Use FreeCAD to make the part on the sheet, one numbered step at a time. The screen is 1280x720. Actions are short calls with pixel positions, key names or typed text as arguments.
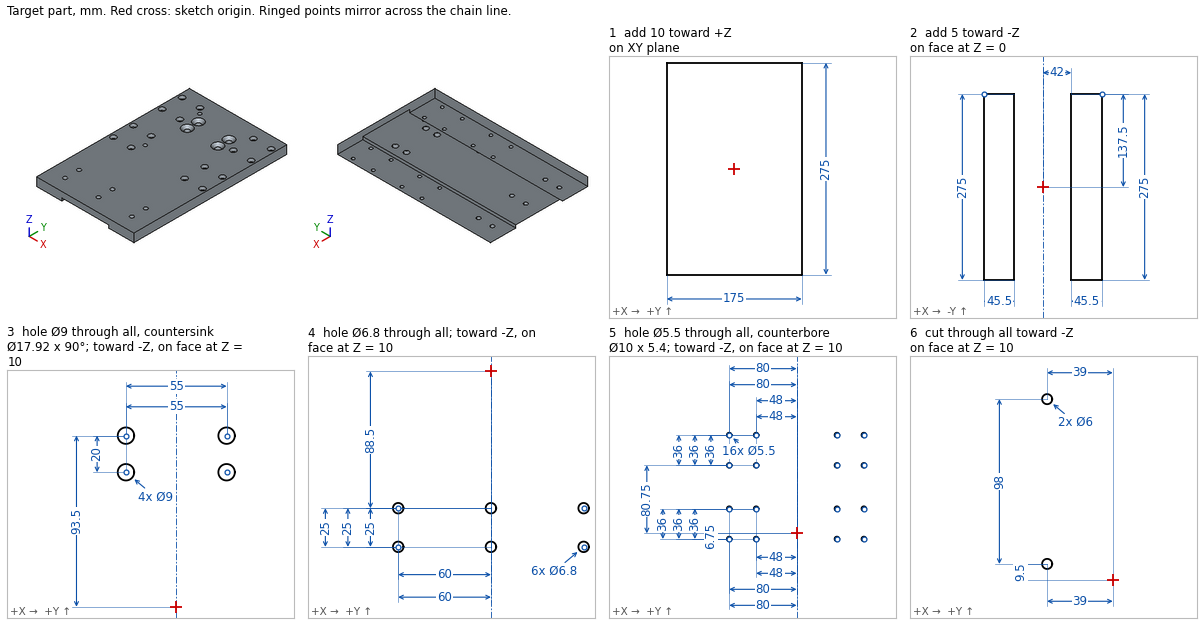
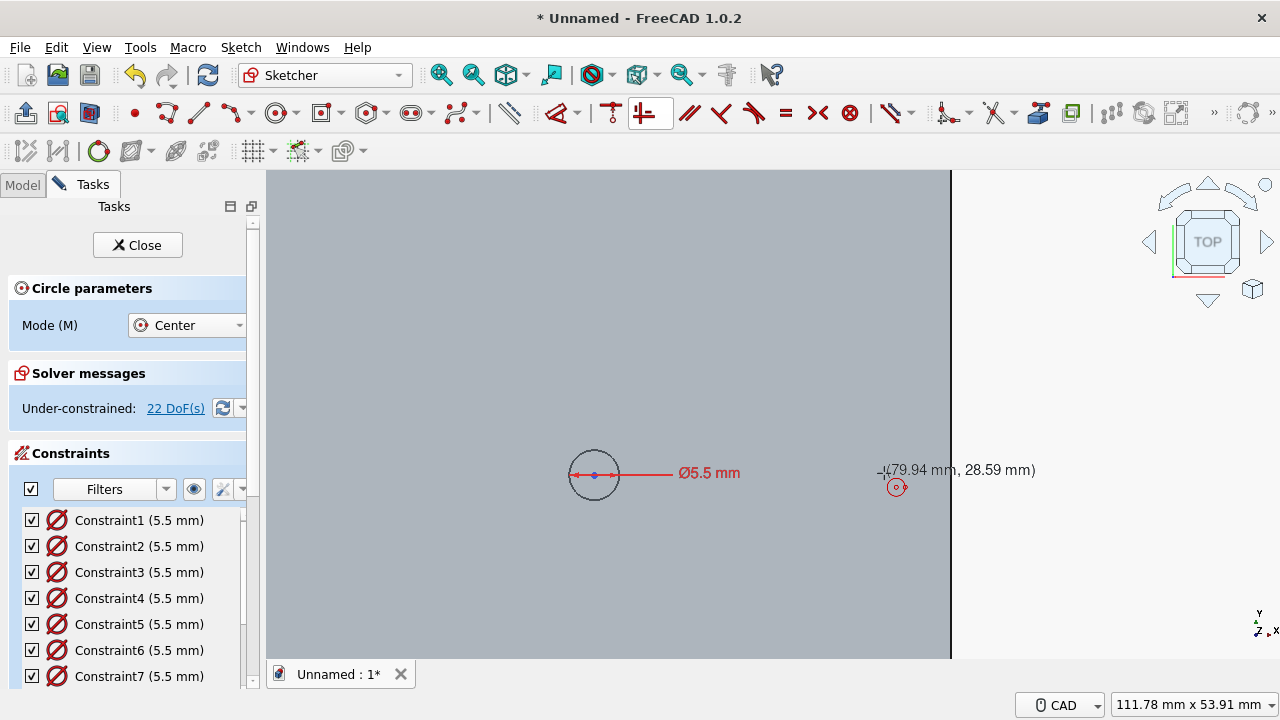
scroll(884, 473, down, 7)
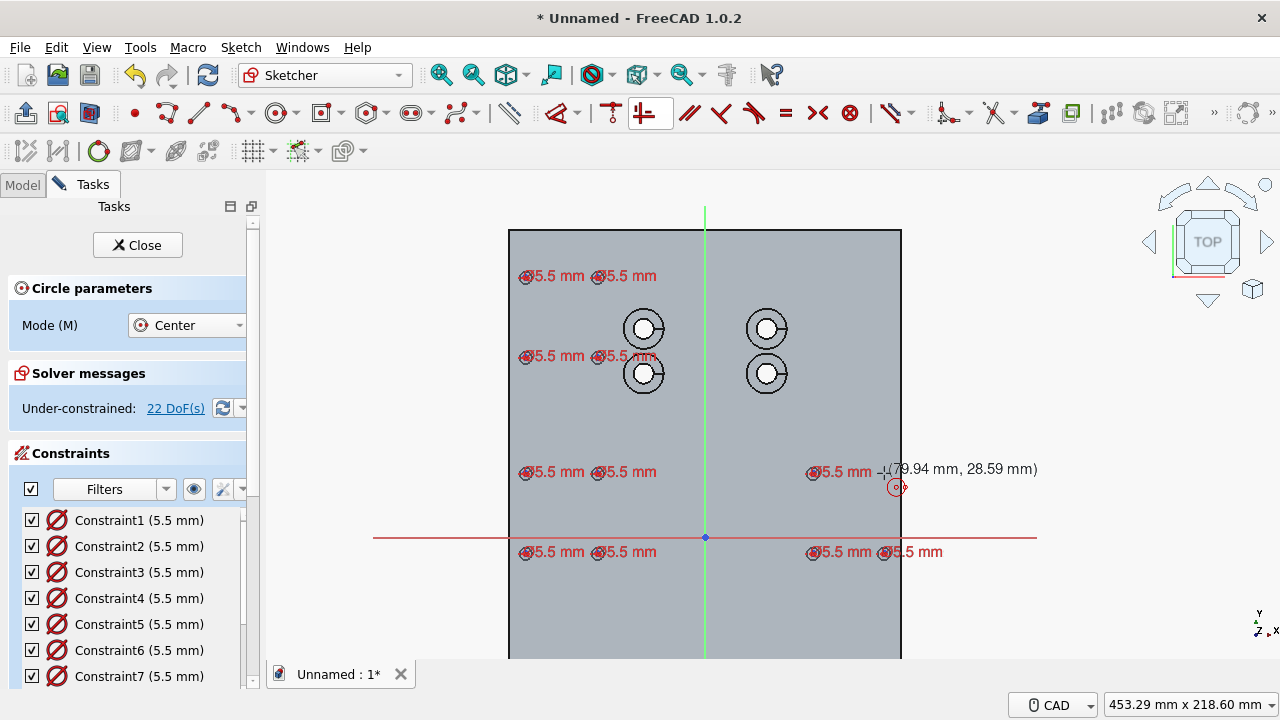
click(884, 473)
move(888, 468)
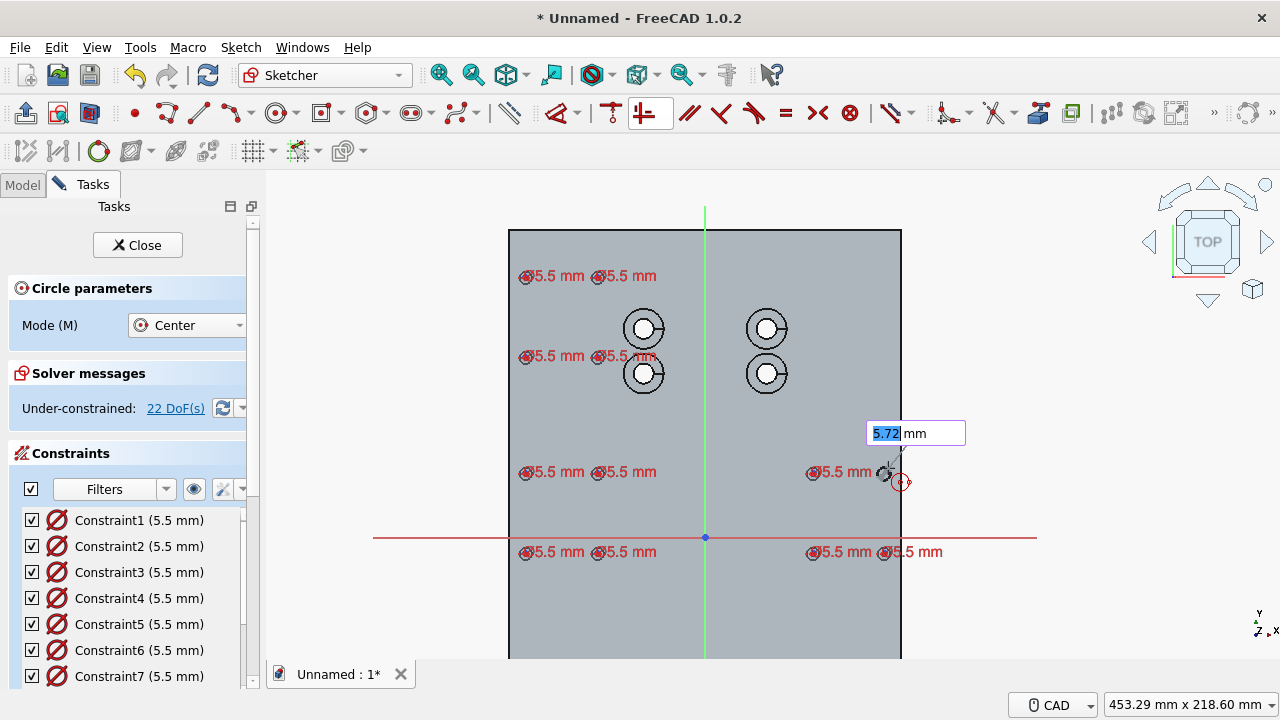
text(5.5)
key(Return)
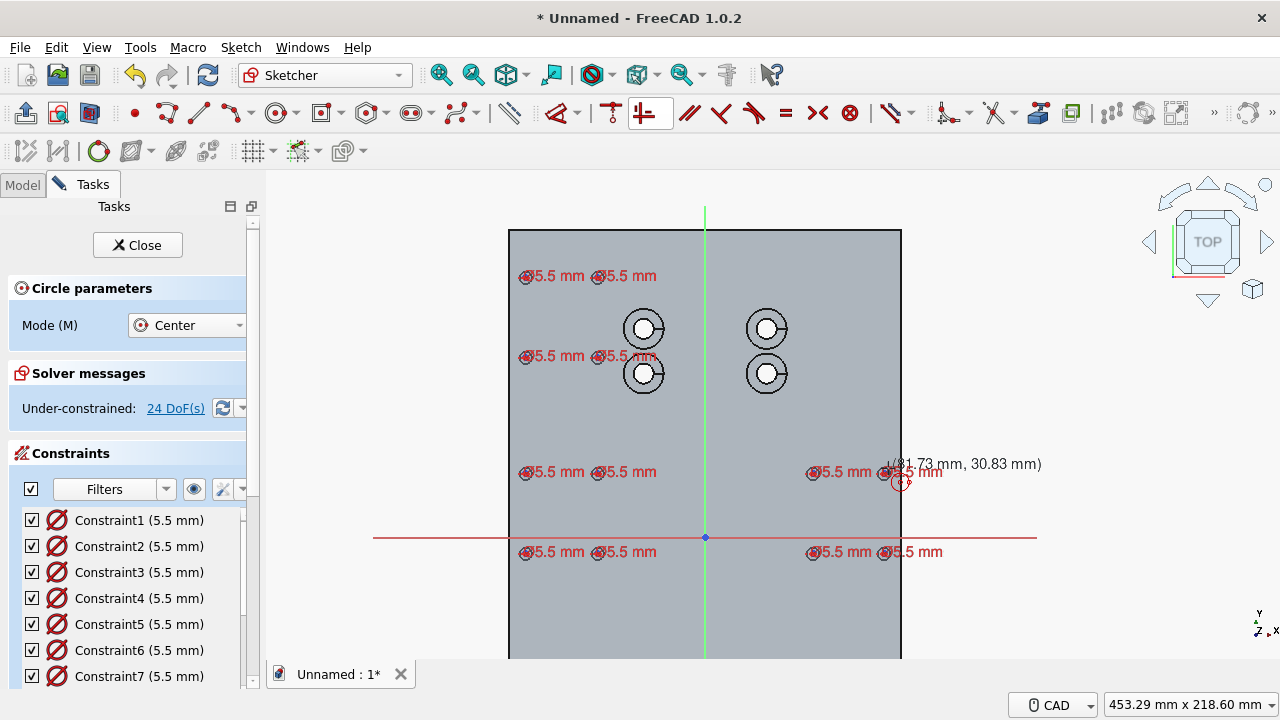
scroll(813, 357, up, 7)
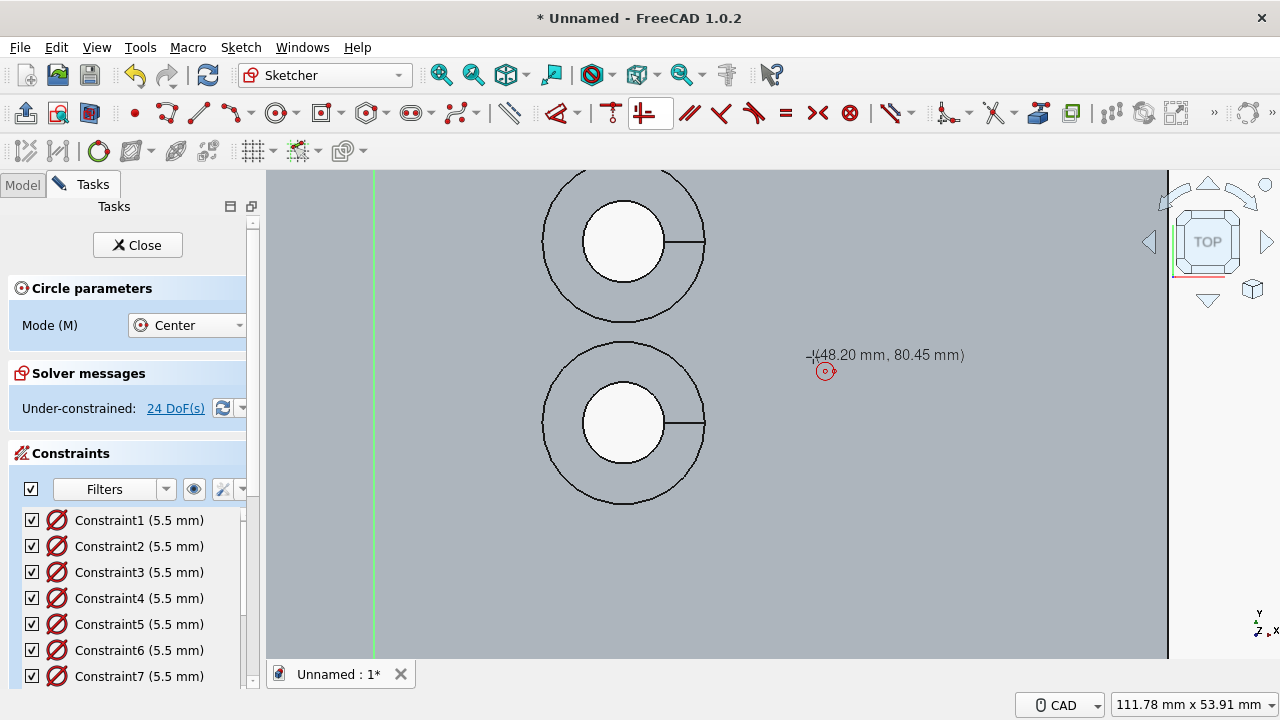
scroll(813, 357, down, 7)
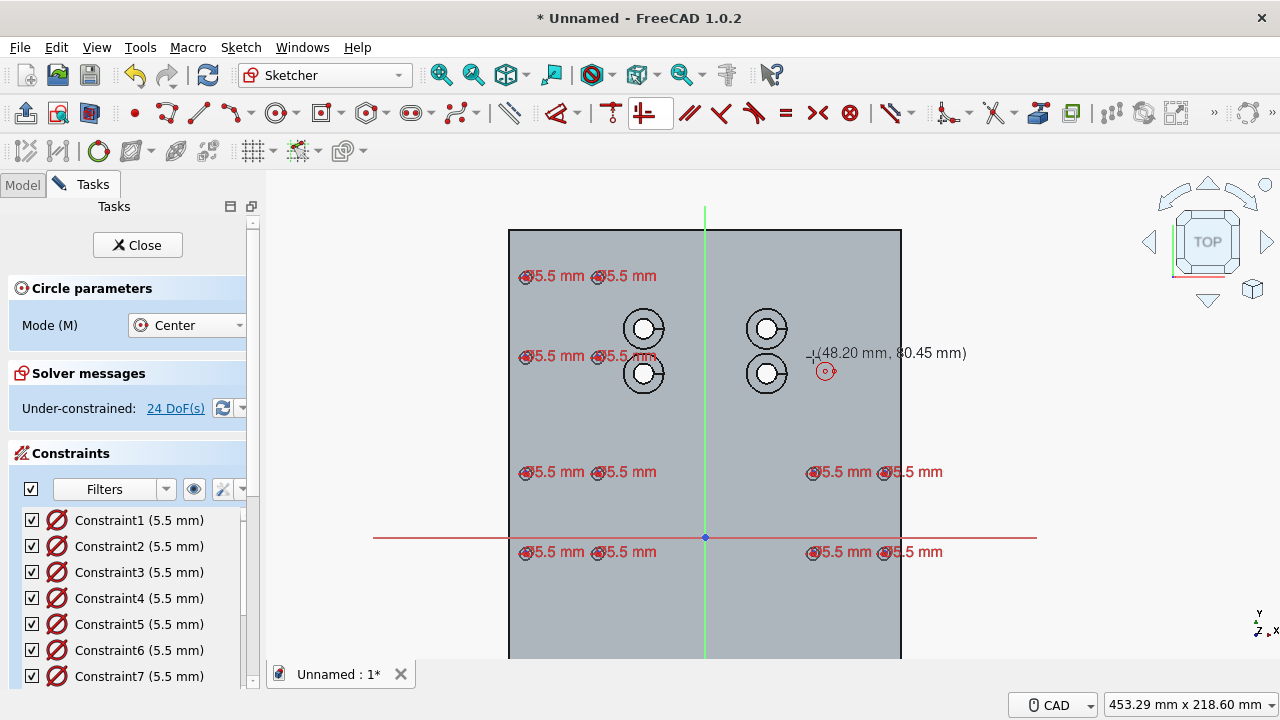
click(813, 357)
move(817, 353)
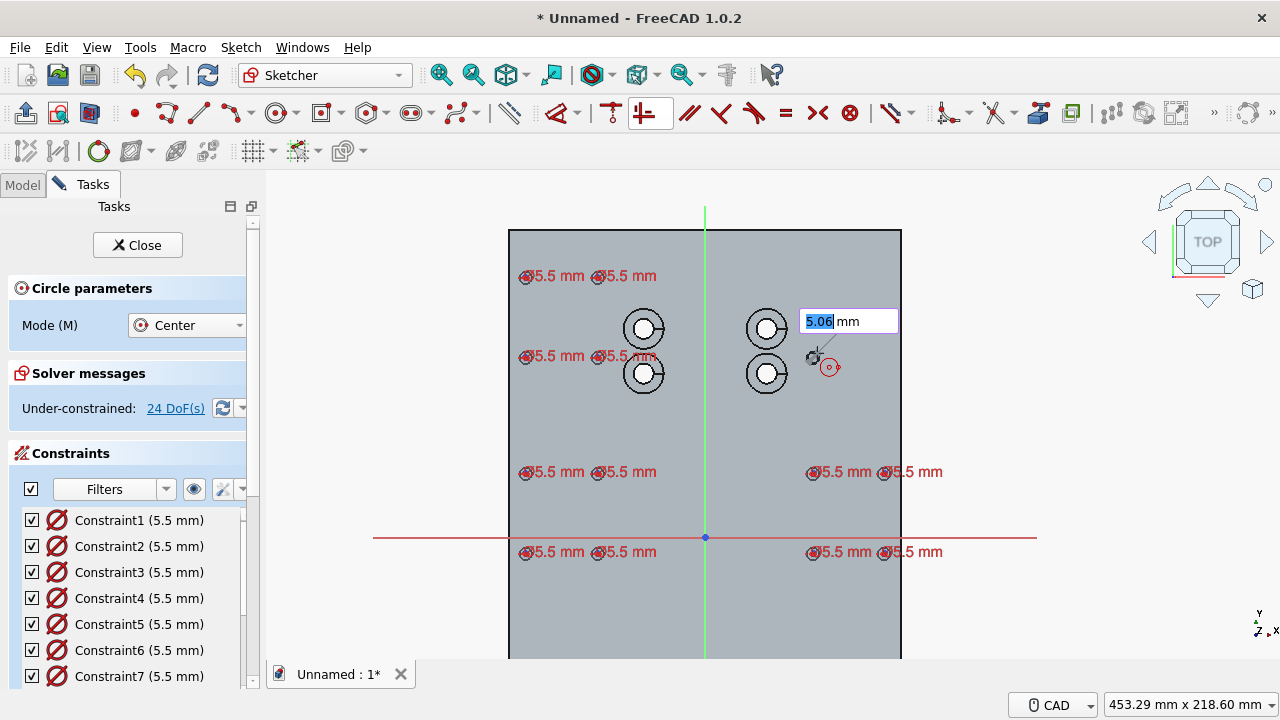
text(5.5)
key(Return)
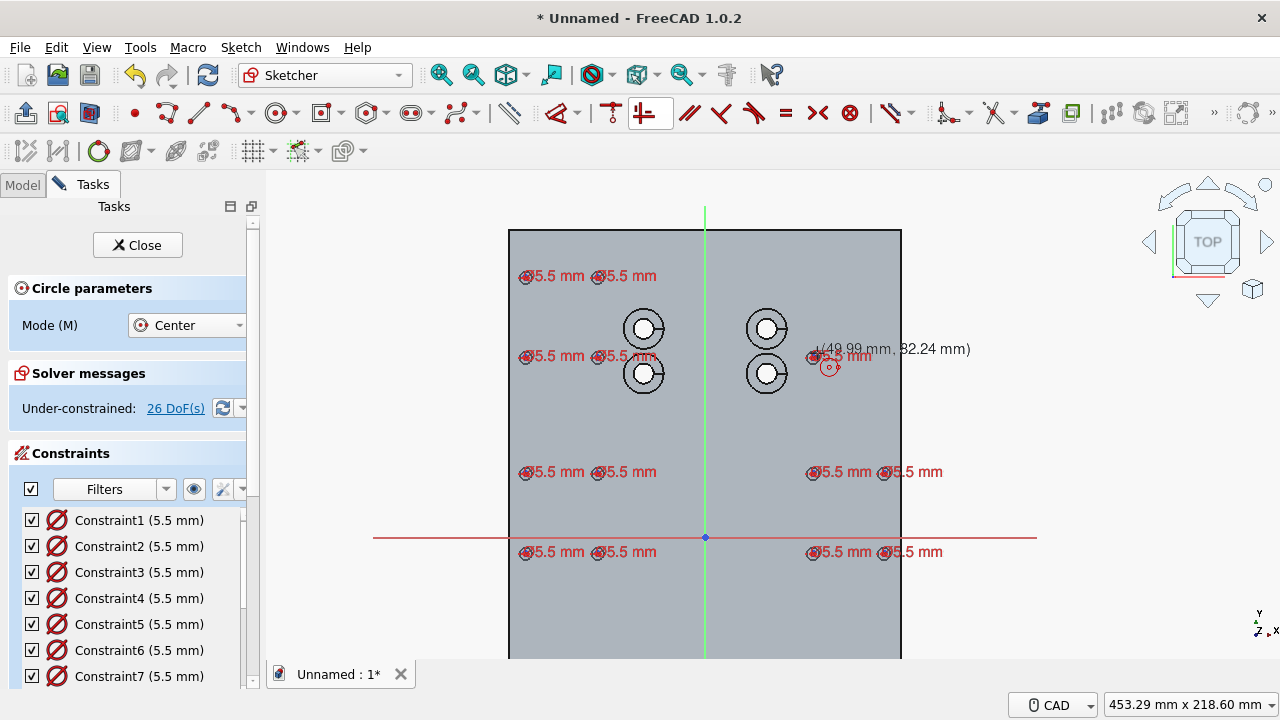
scroll(884, 357, up, 7)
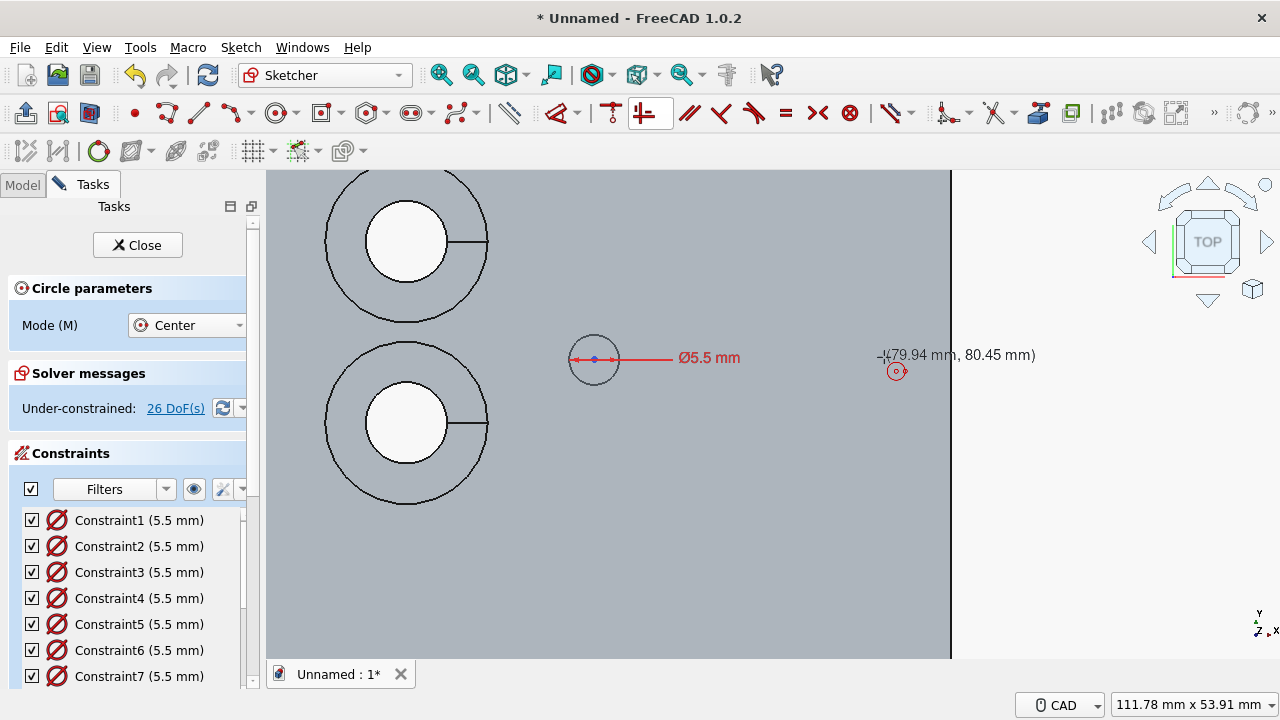
scroll(884, 357, down, 7)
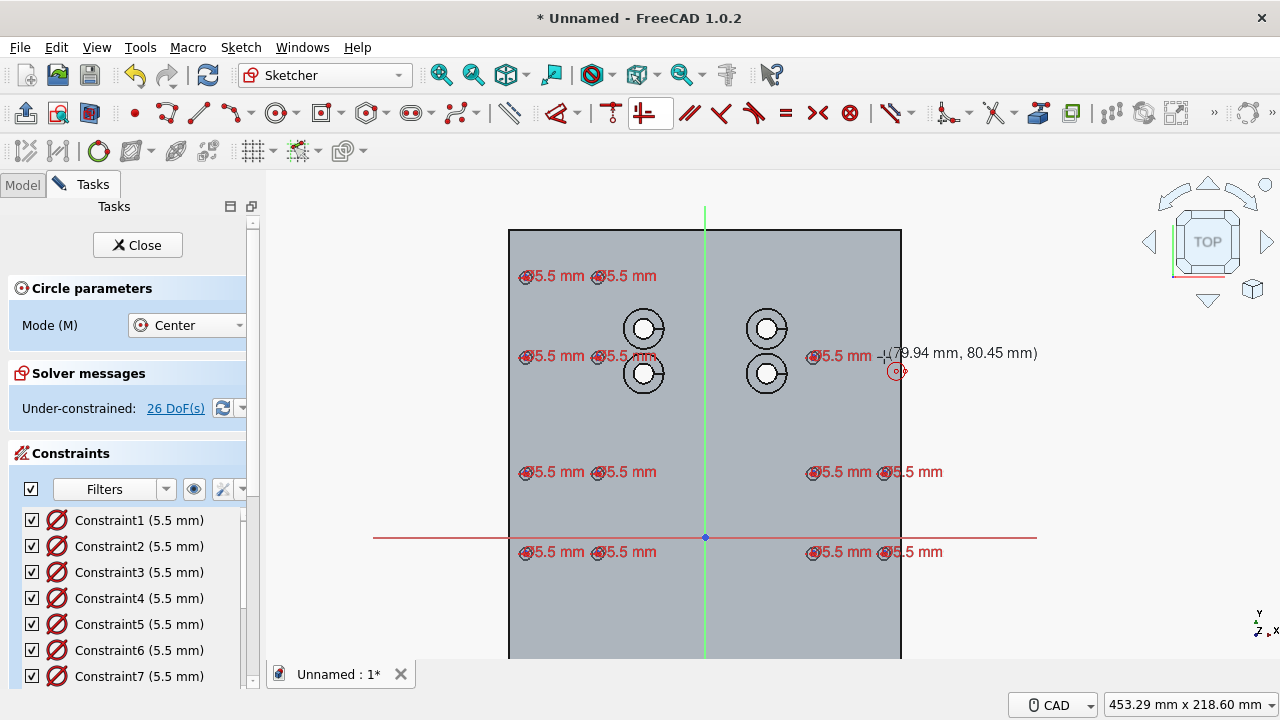
click(884, 357)
move(888, 353)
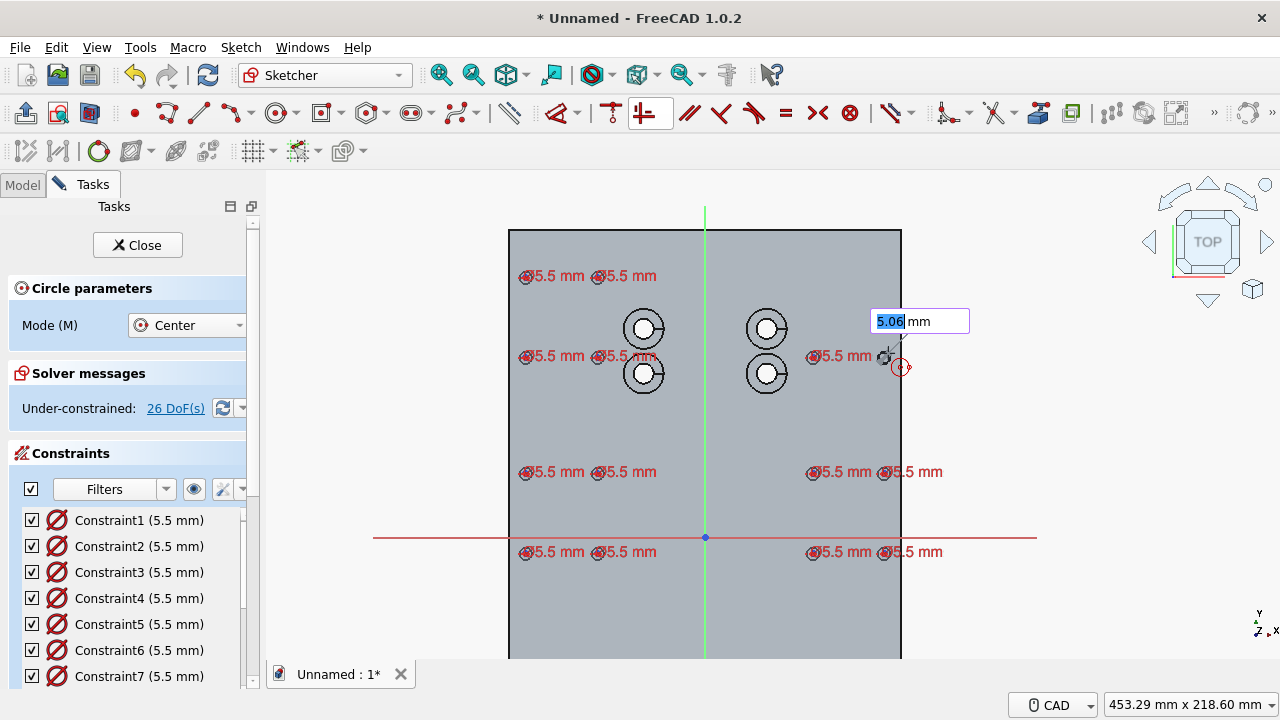
text(5.5)
key(Return)